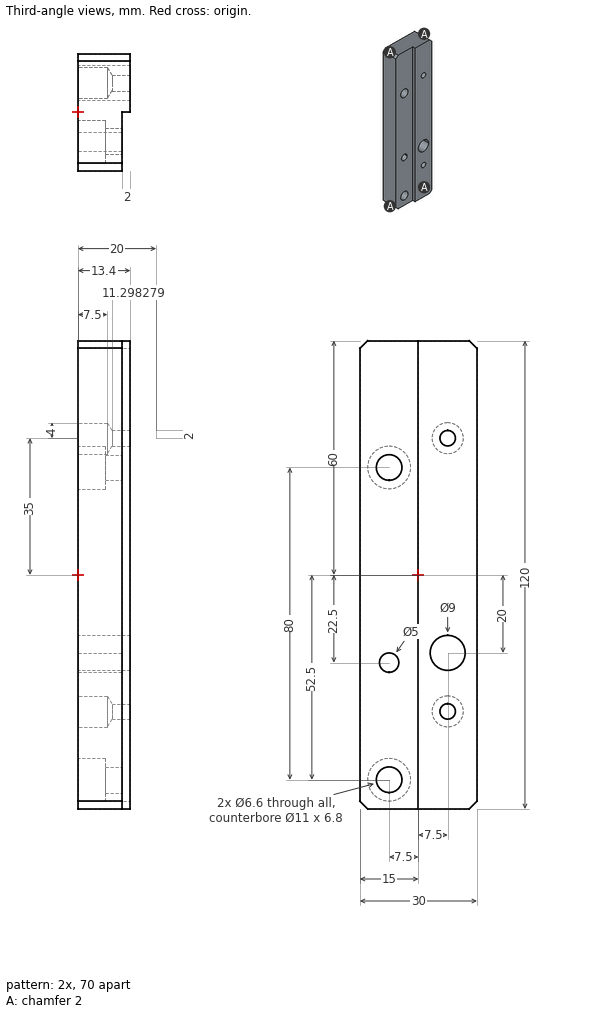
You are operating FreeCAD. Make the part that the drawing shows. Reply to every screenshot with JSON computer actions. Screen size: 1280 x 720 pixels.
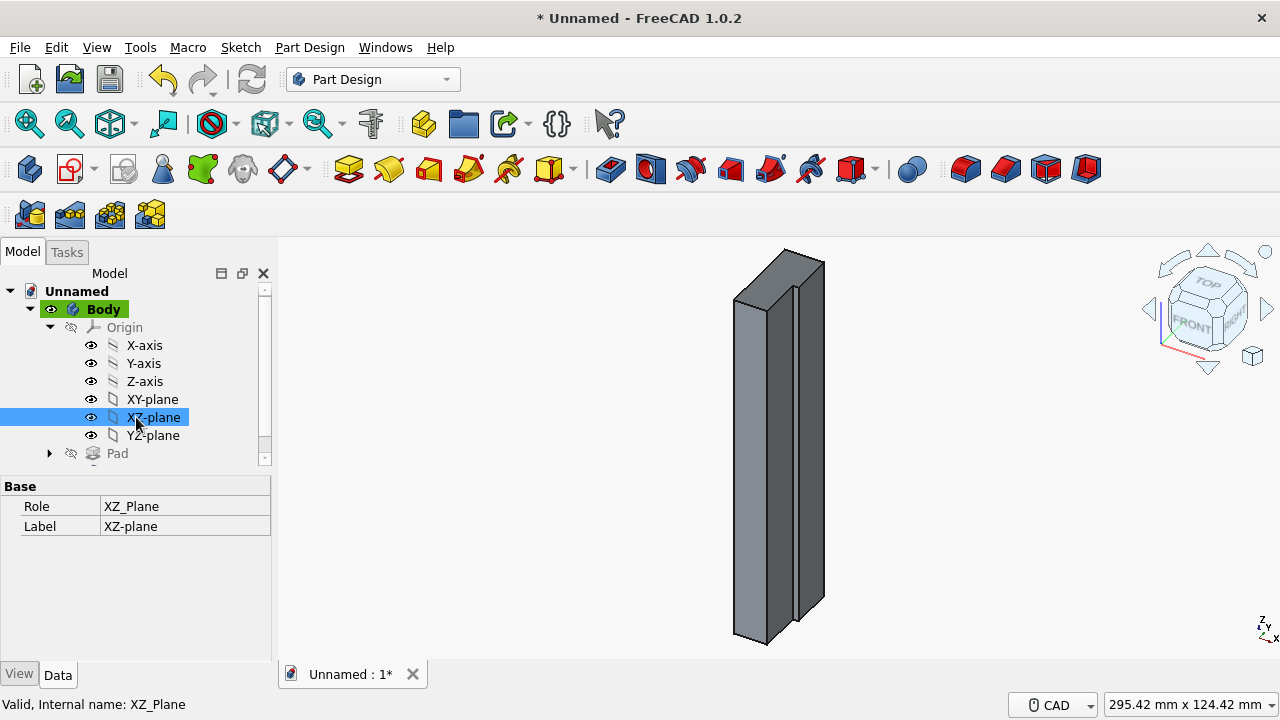
{"action": "left_click", "coordinate": [284, 170]}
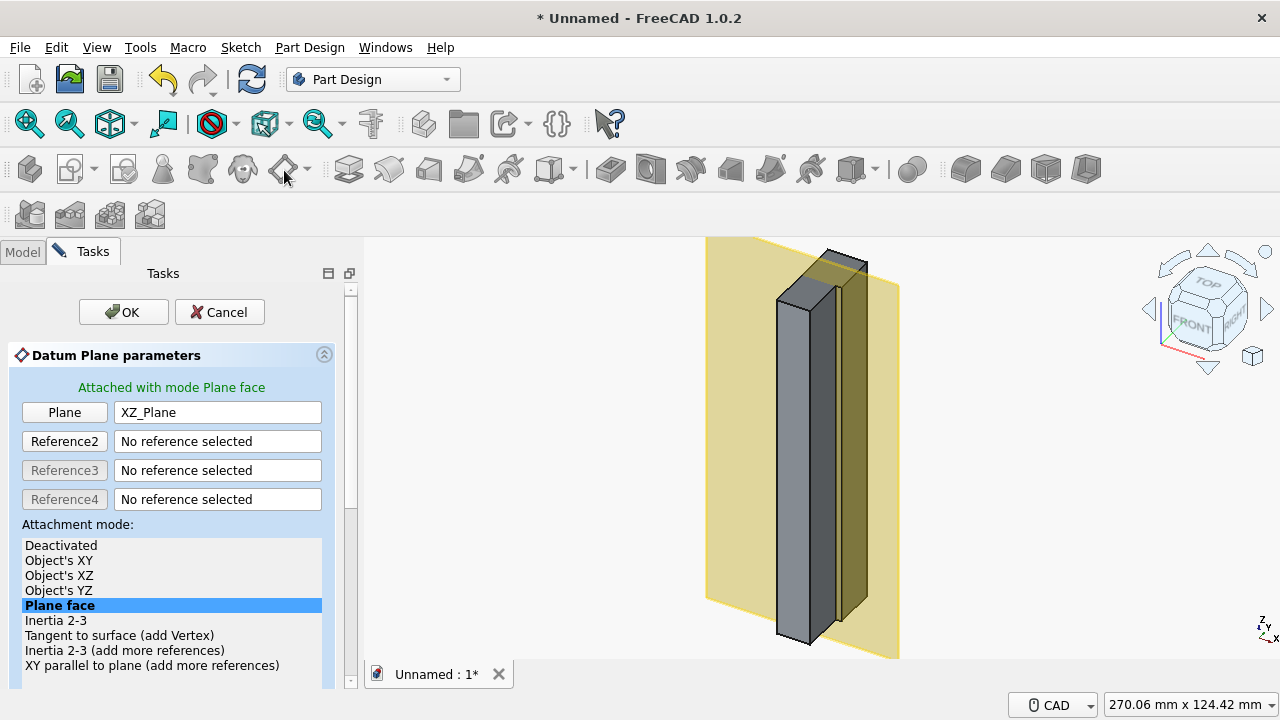
{"action": "scroll", "coordinate": [351, 486], "scroll_direction": "down", "scroll_amount": 4}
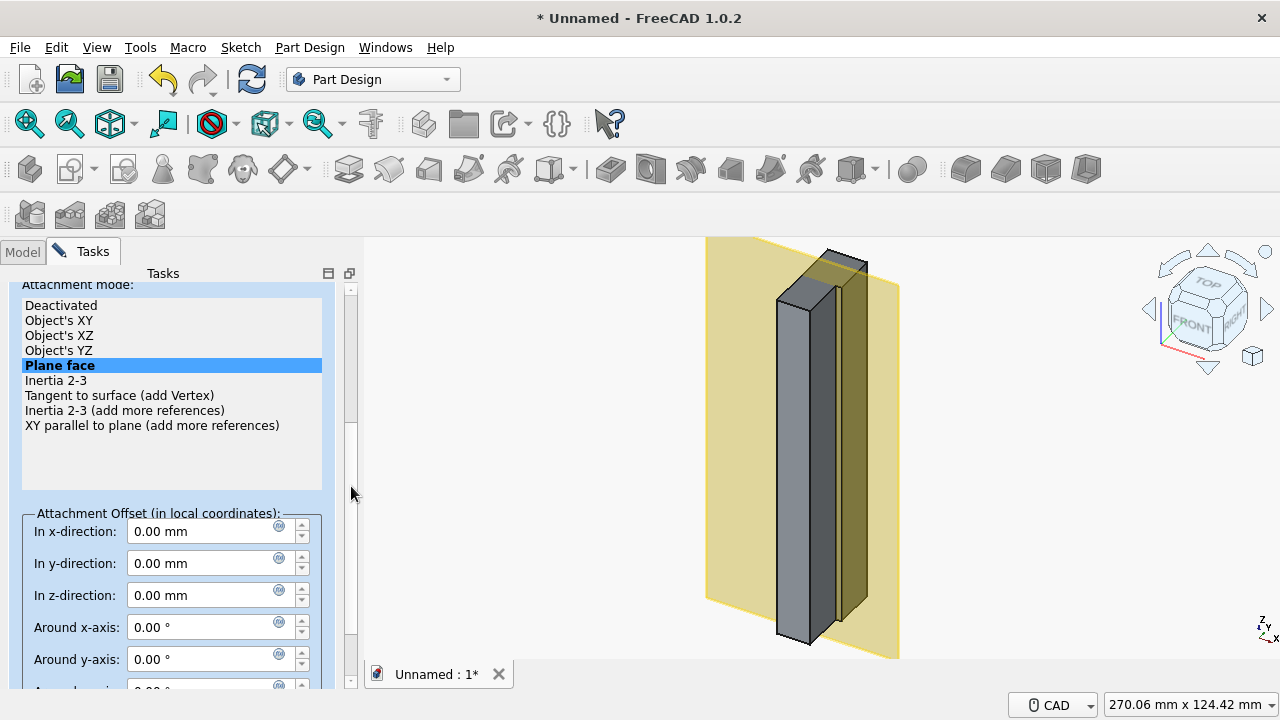
{"action": "triple_click", "coordinate": [210, 595]}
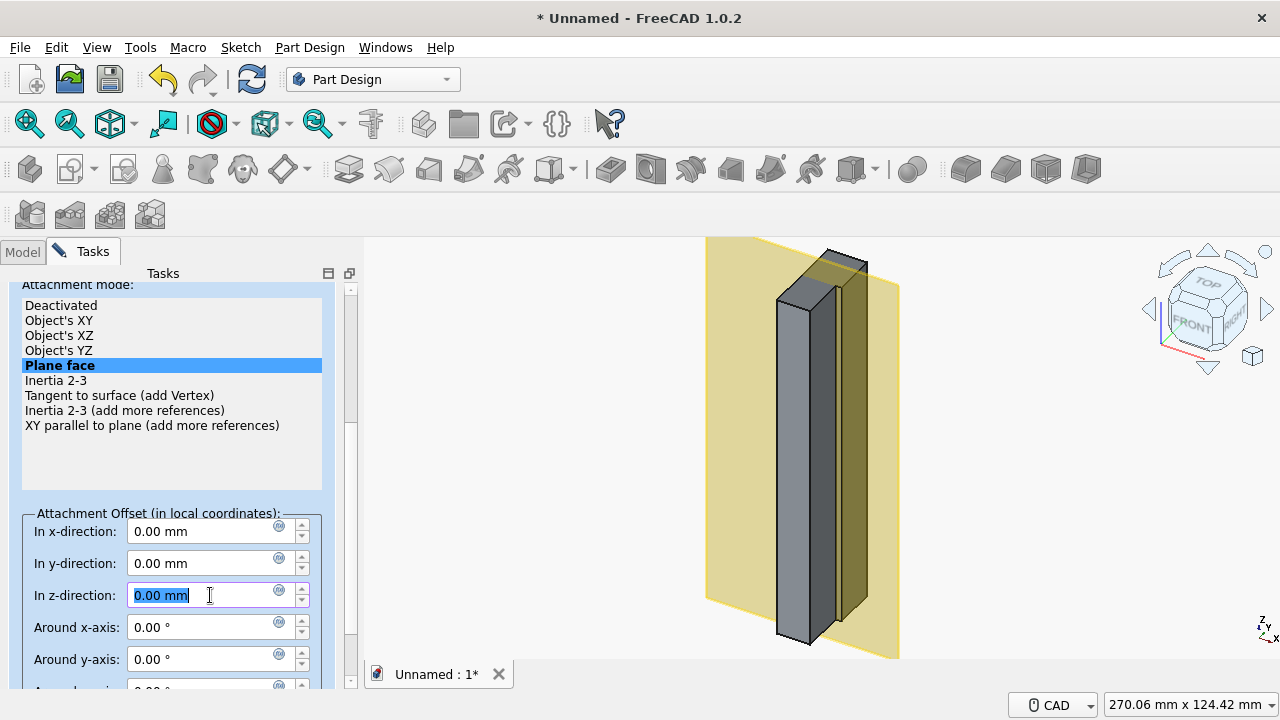
{"action": "type", "text": "-7.5"}
{"action": "key", "text": "Tab"}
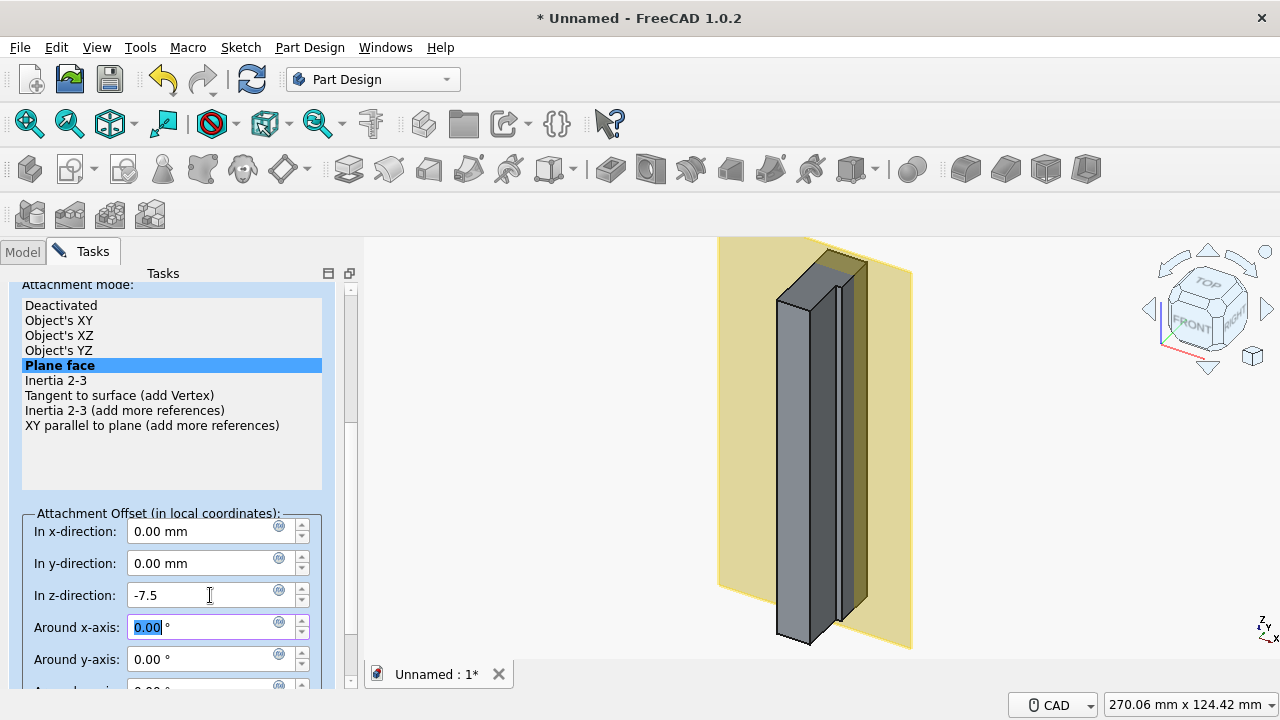
{"action": "scroll", "coordinate": [351, 486], "scroll_direction": "up", "scroll_amount": 5}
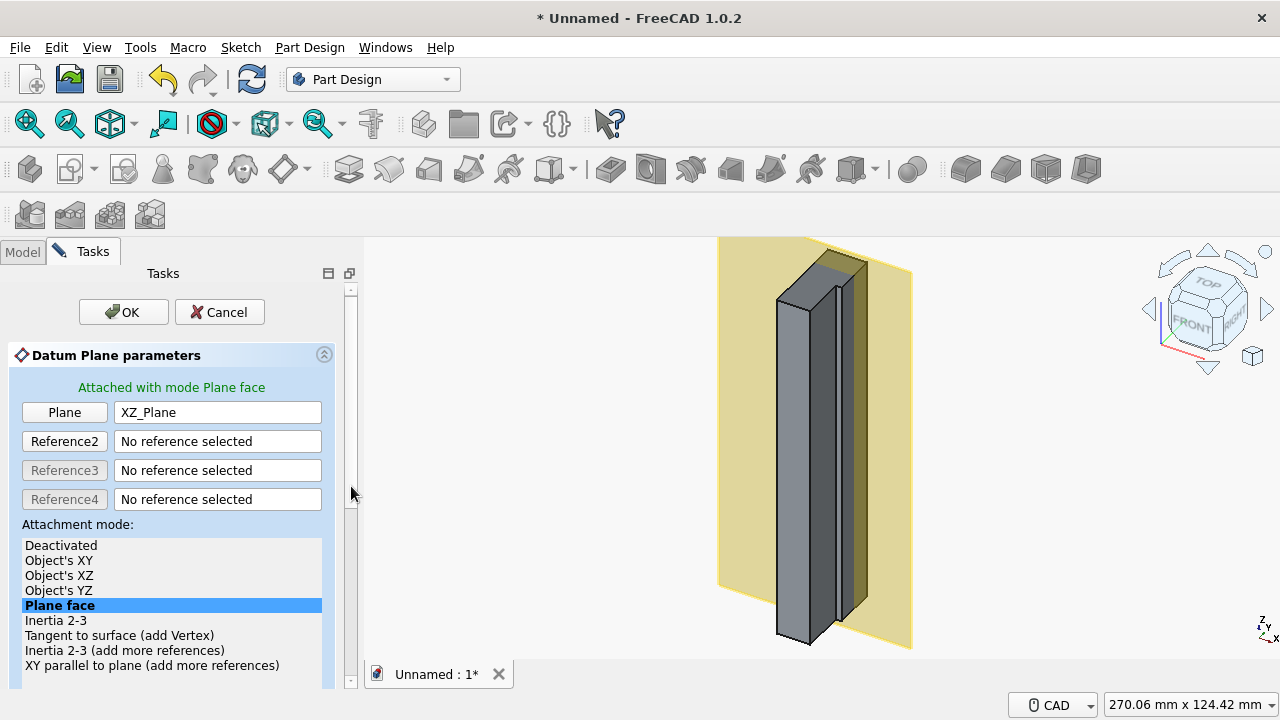
{"action": "left_click", "coordinate": [124, 312]}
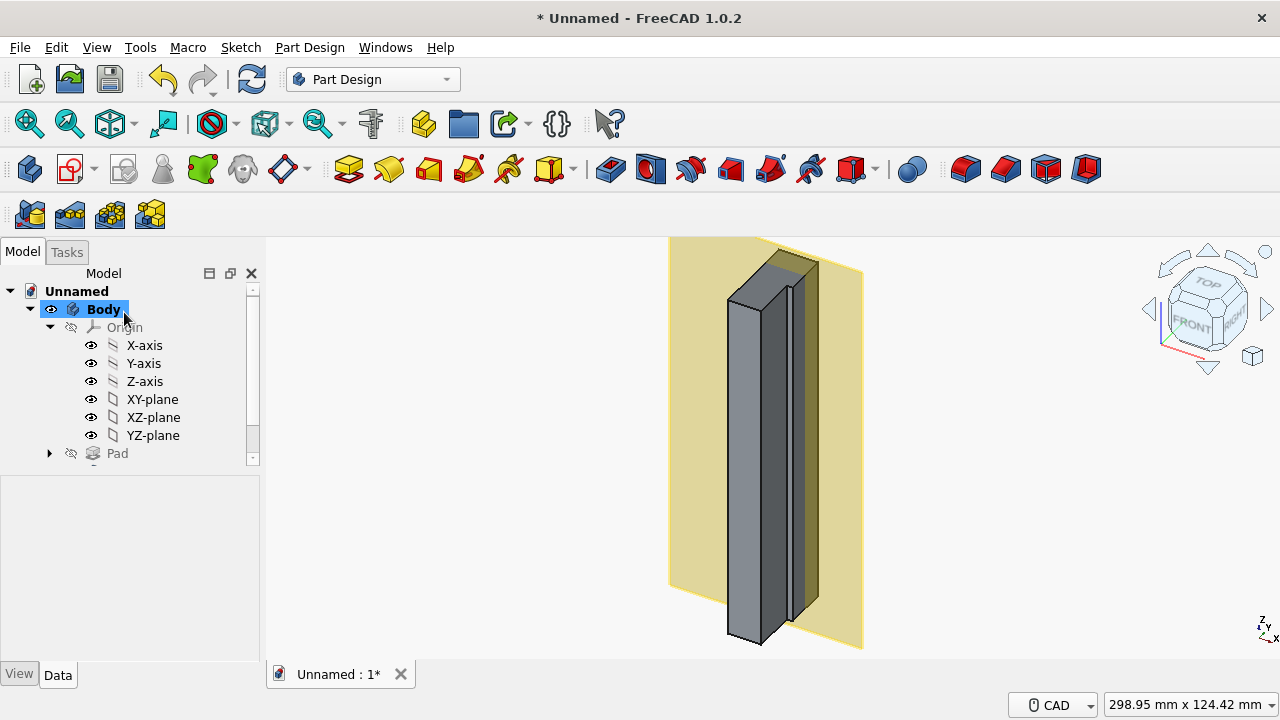
{"action": "scroll", "coordinate": [100, 377], "scroll_direction": "down", "scroll_amount": 3}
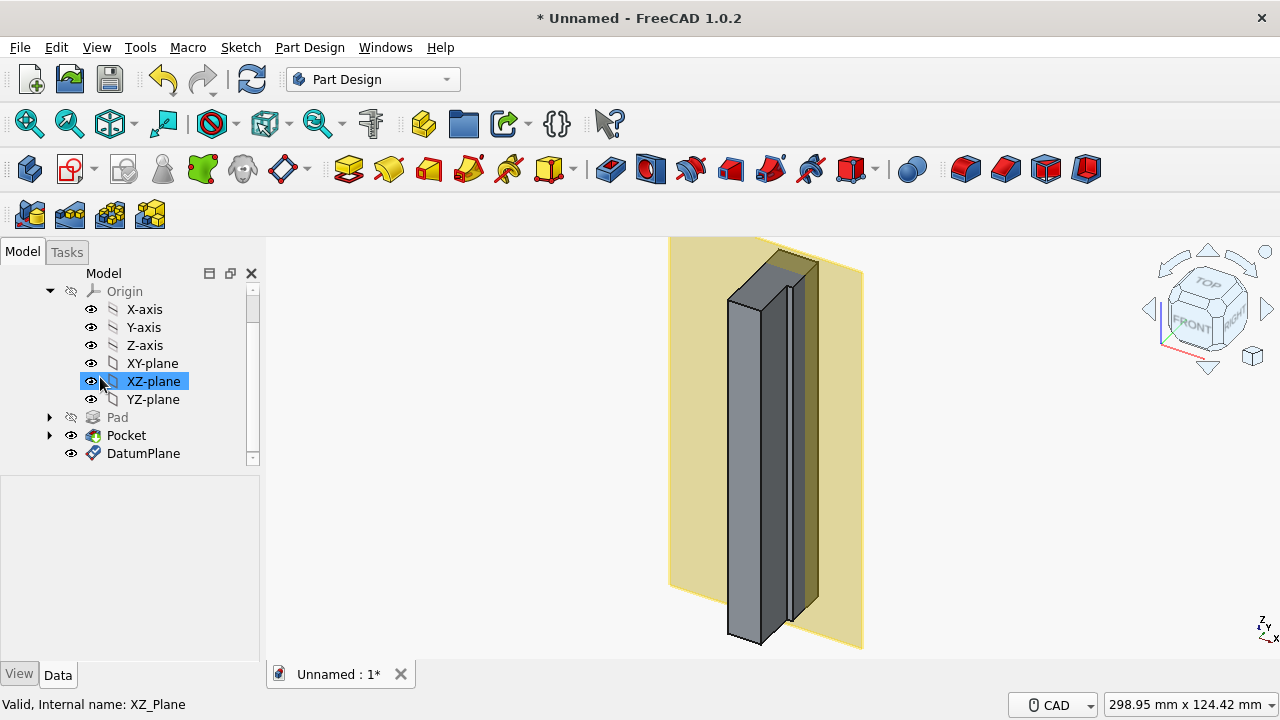
{"action": "left_click", "coordinate": [116, 453]}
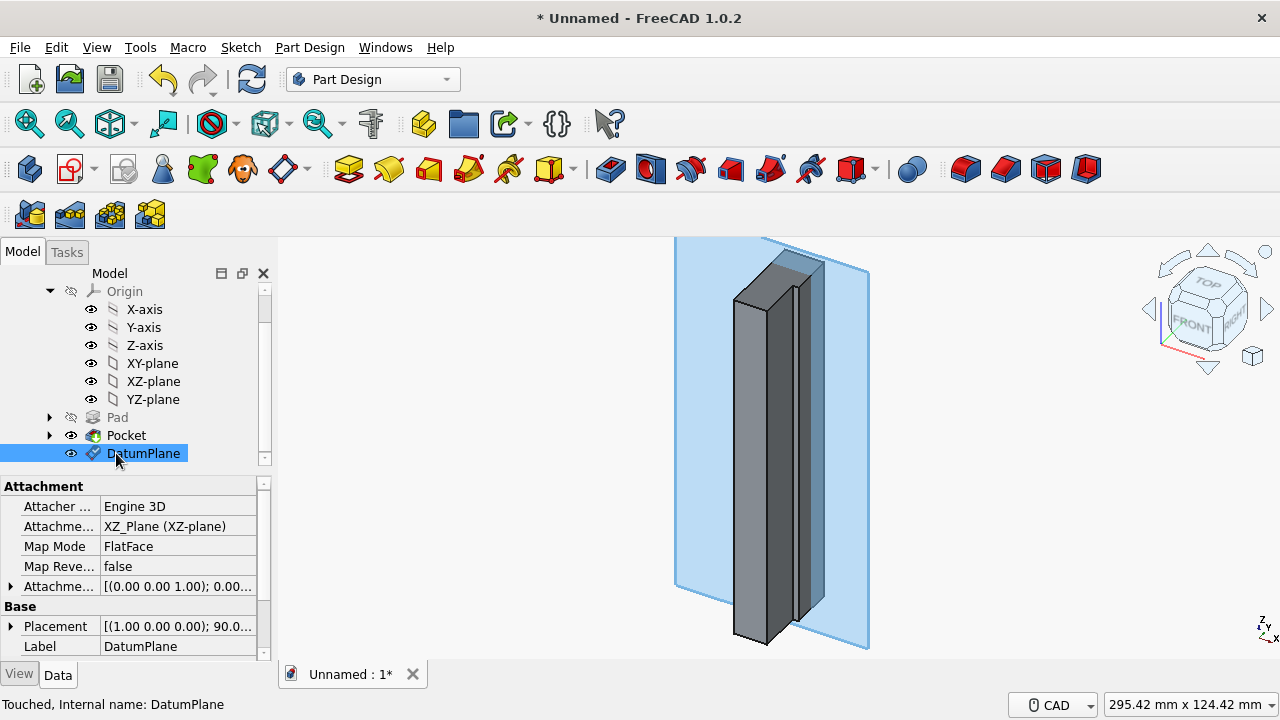
{"action": "left_click", "coordinate": [70, 170]}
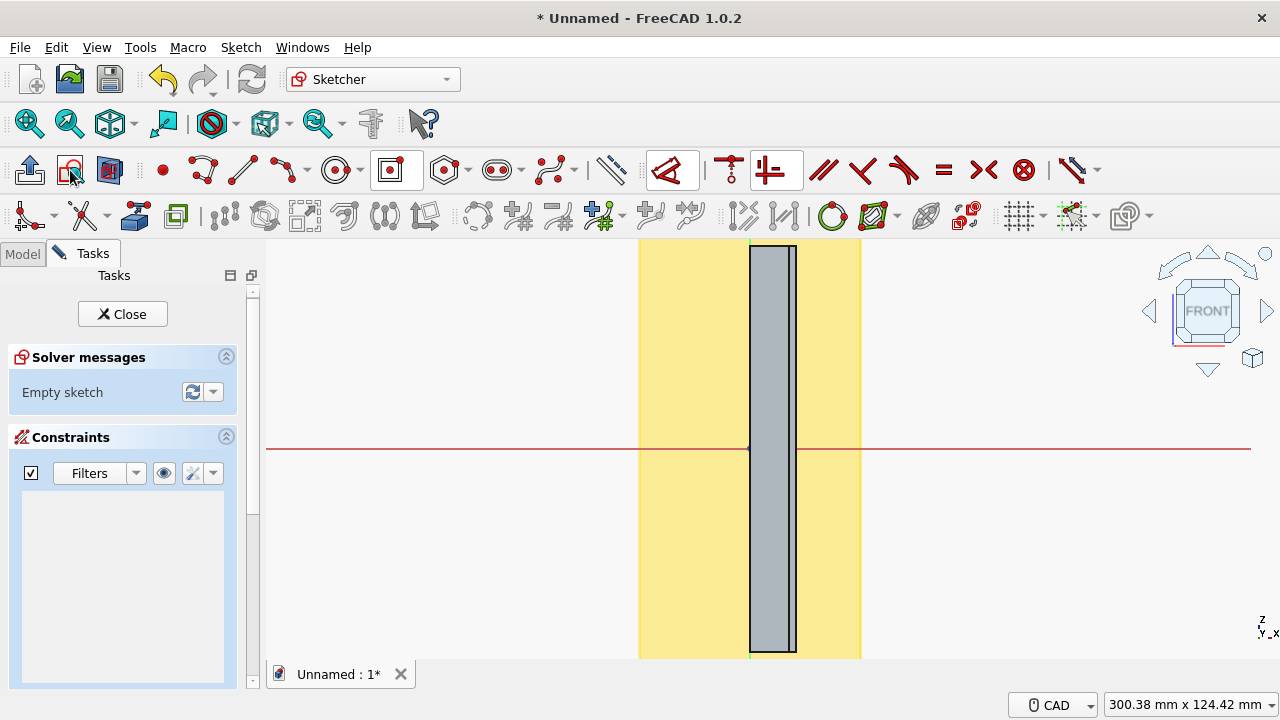
{"action": "left_click", "coordinate": [110, 170]}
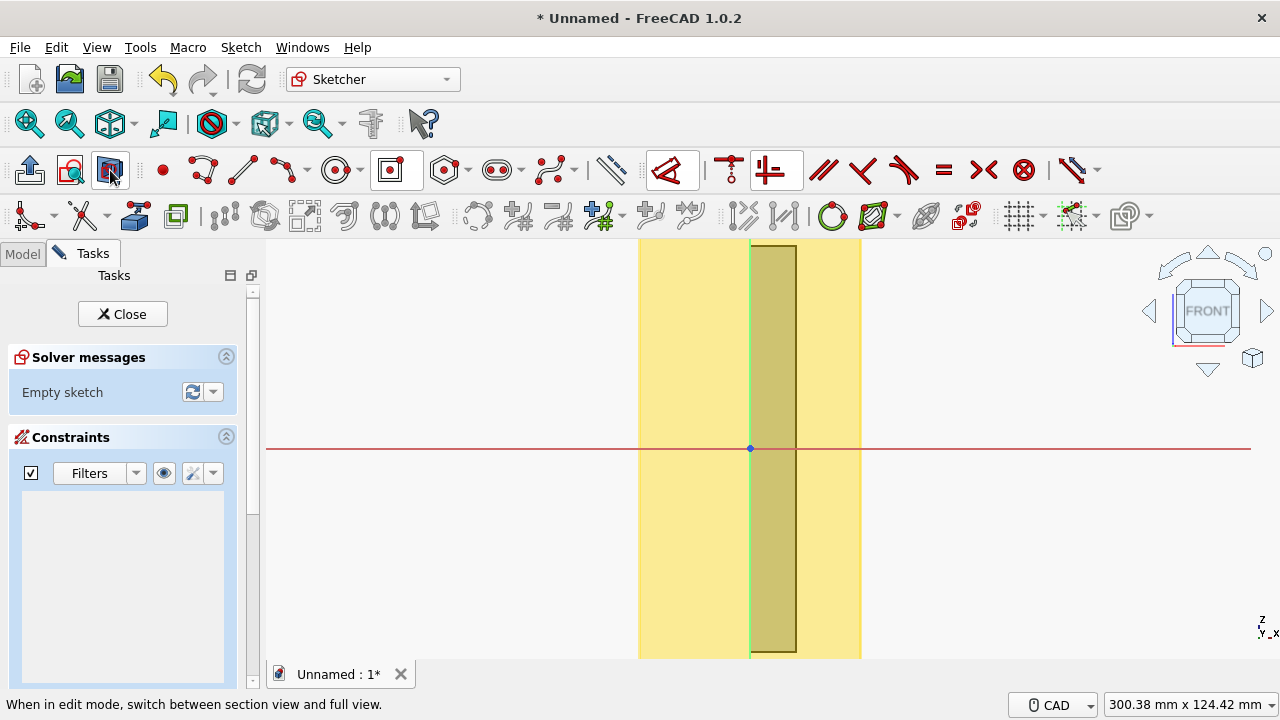
{"action": "scroll", "coordinate": [911, 303], "scroll_direction": "up", "scroll_amount": 3}